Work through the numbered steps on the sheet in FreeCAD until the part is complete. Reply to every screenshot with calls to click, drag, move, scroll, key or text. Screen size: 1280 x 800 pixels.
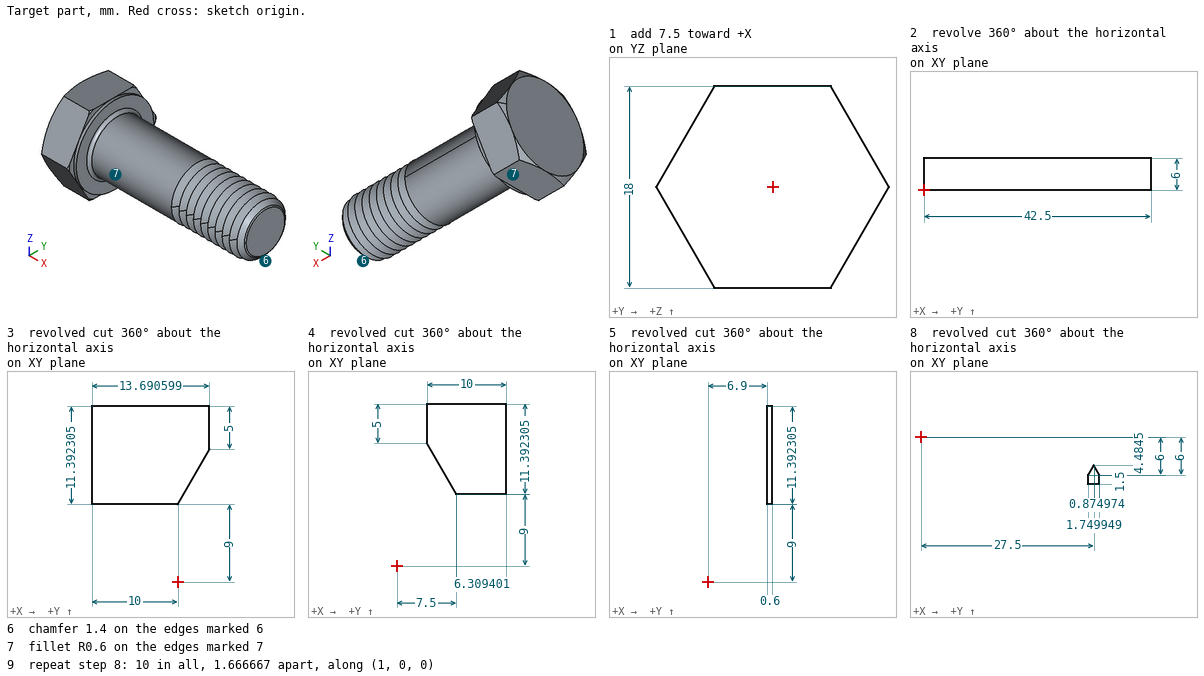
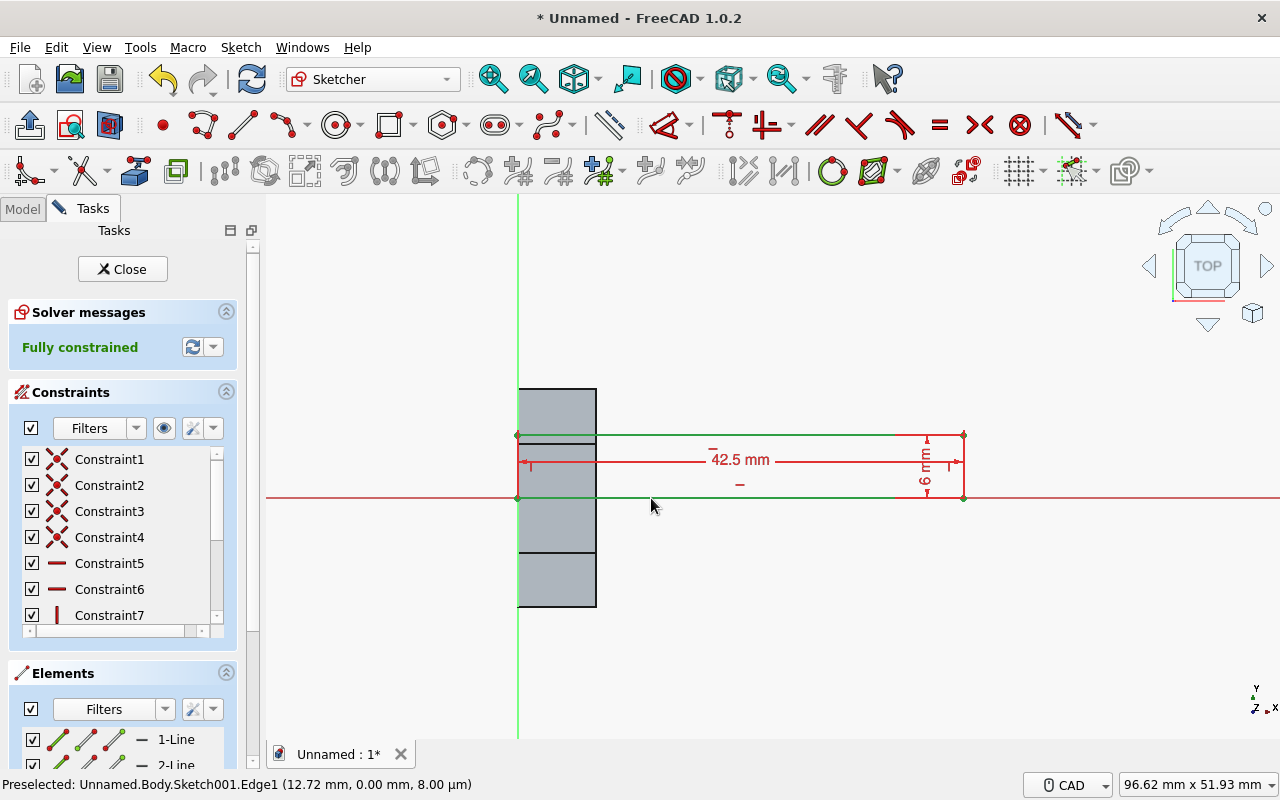
click(123, 269)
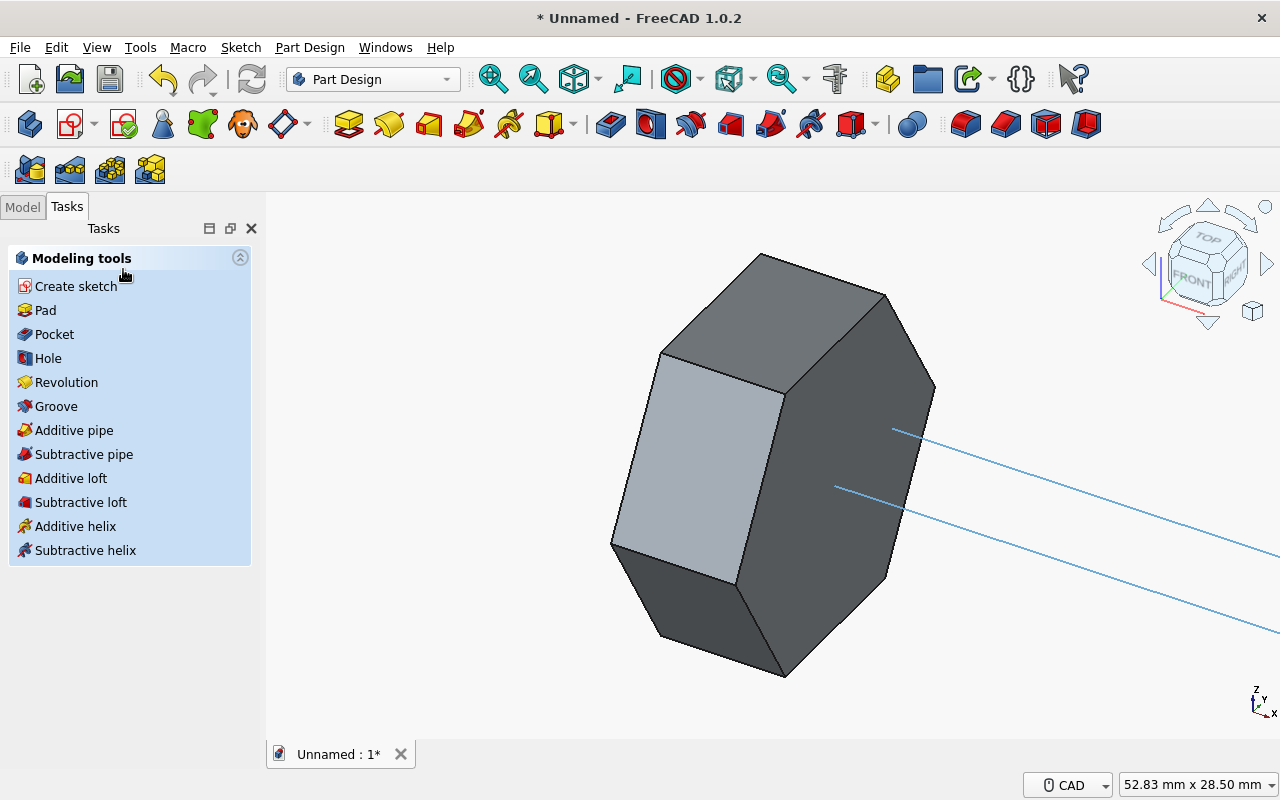
click(390, 124)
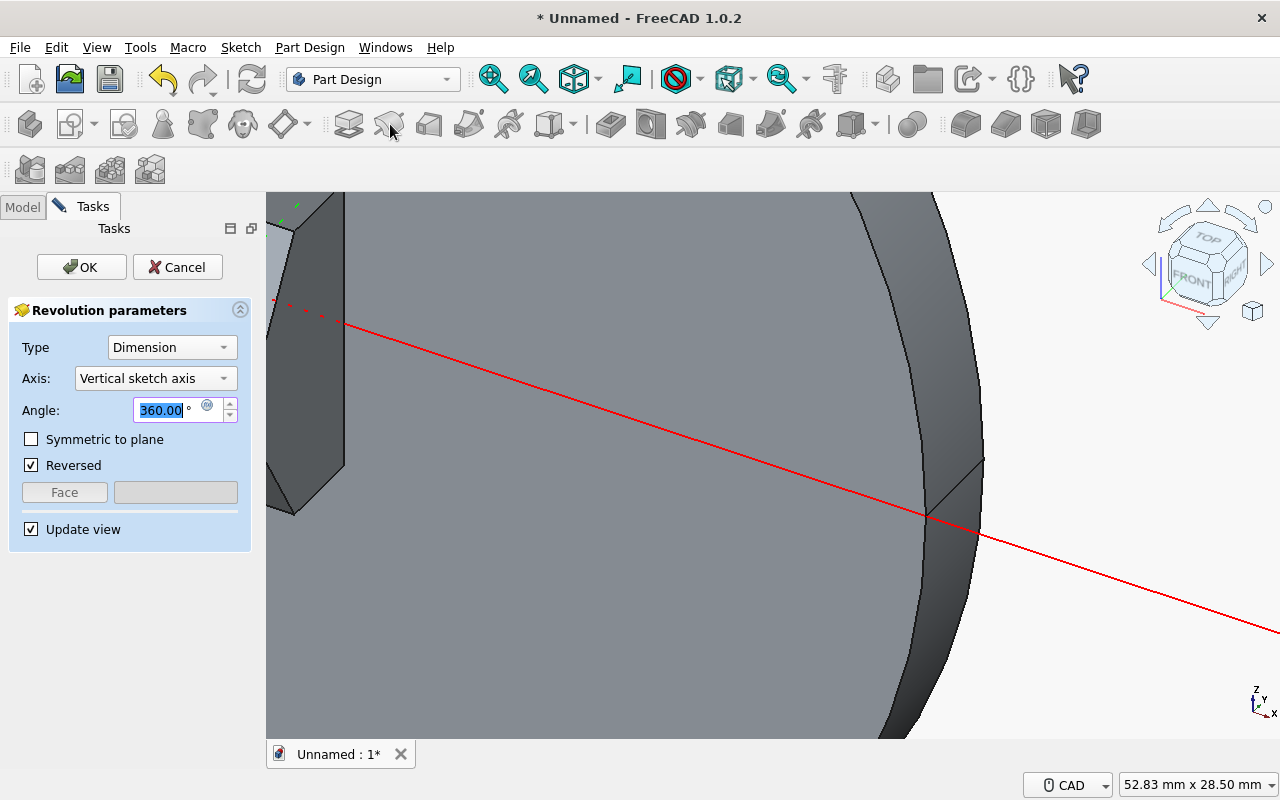
click(156, 378)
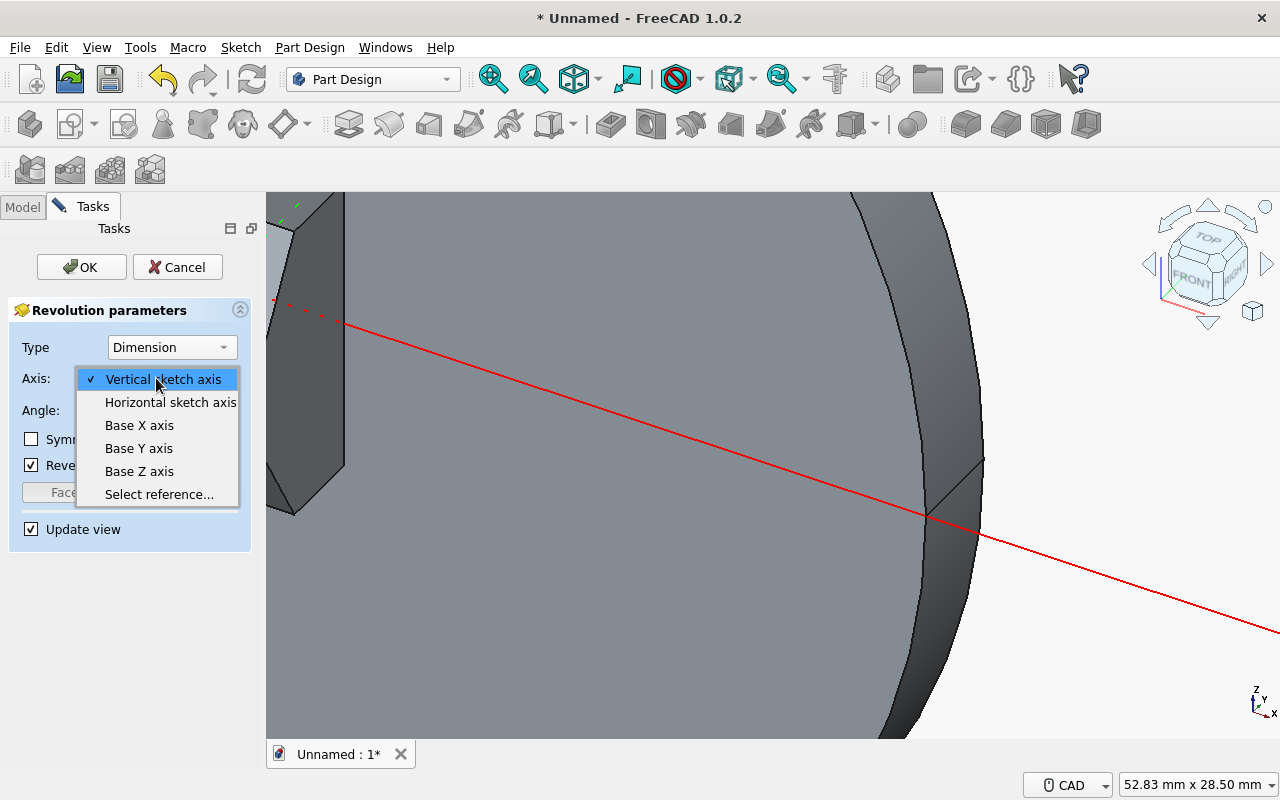
click(156, 402)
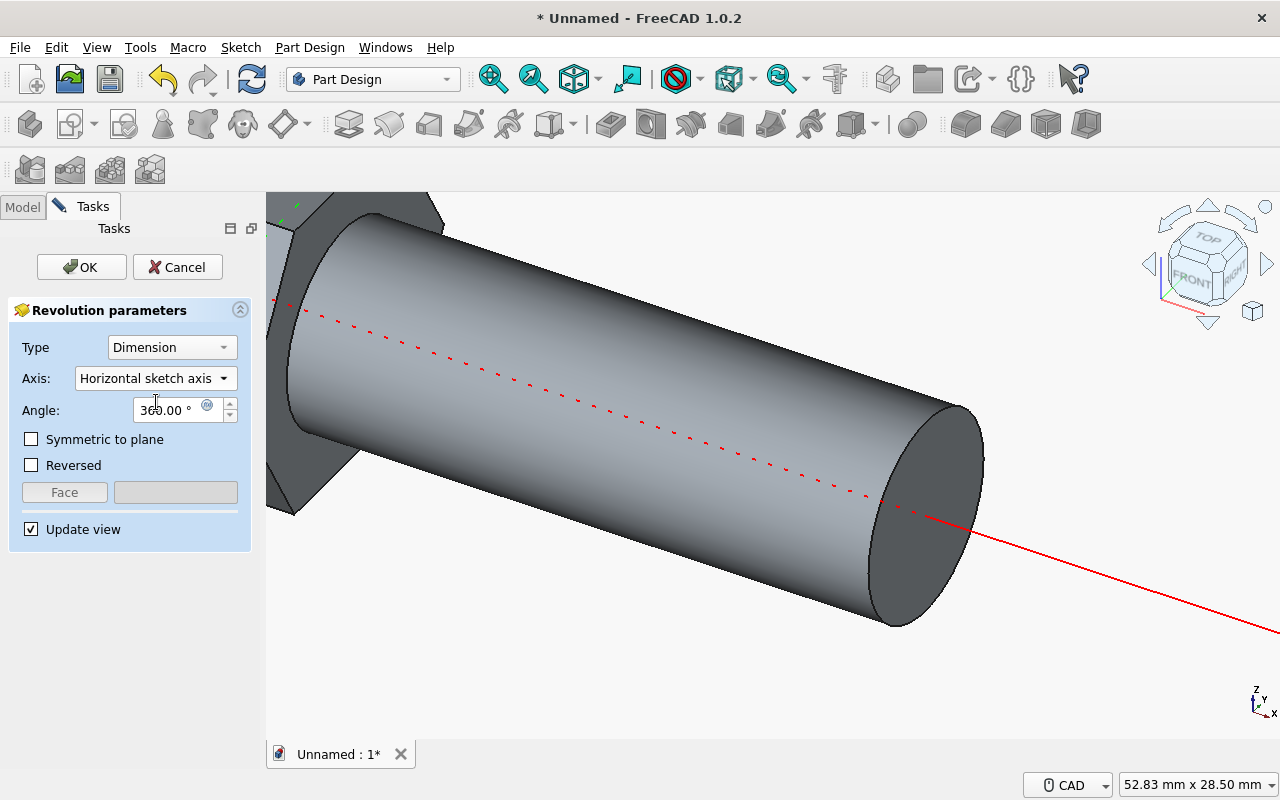
click(82, 267)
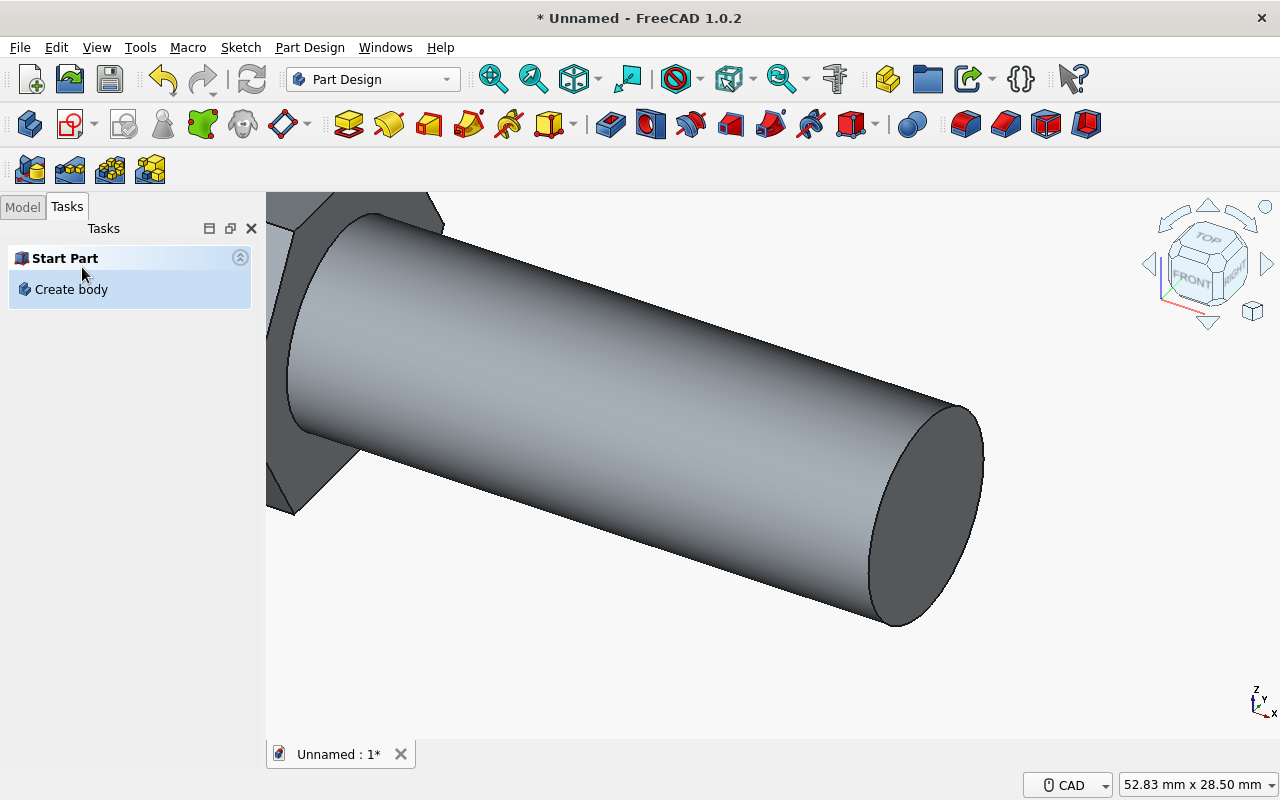
key(v)
key(f)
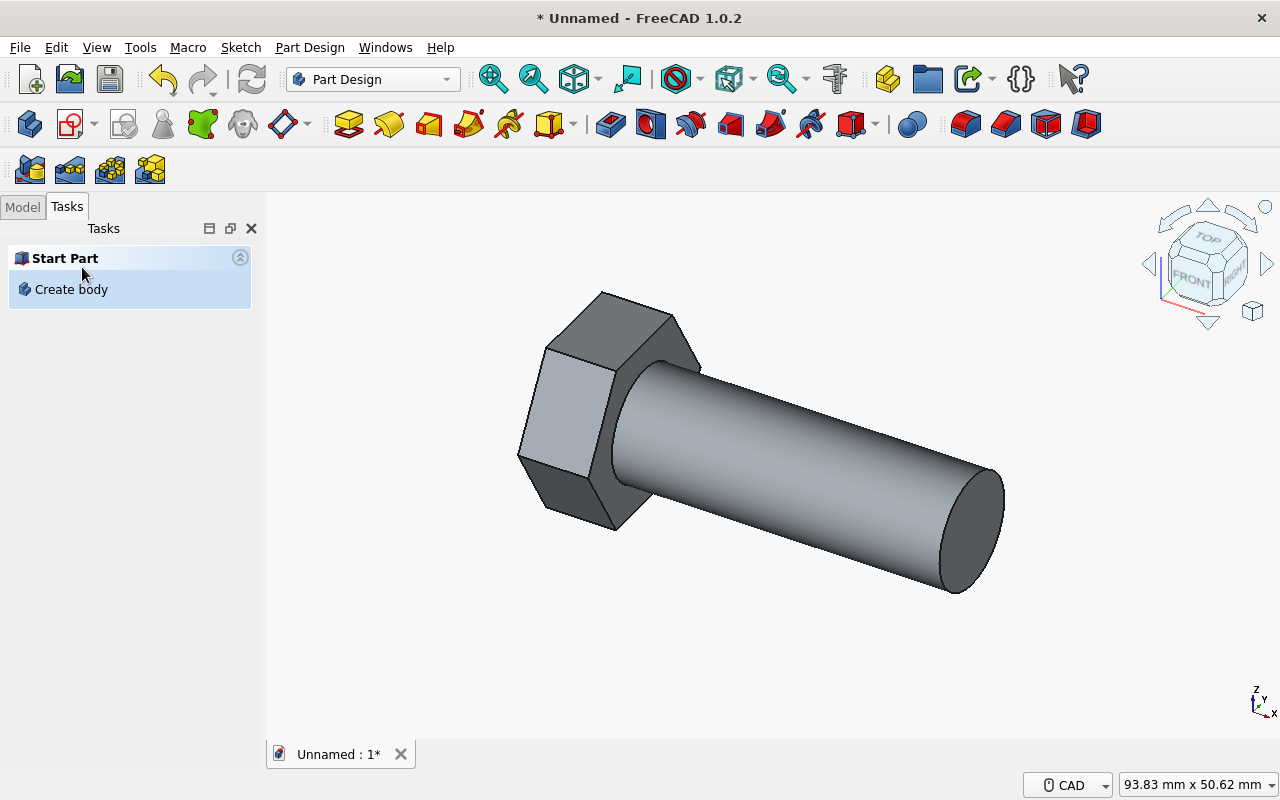
click(70, 124)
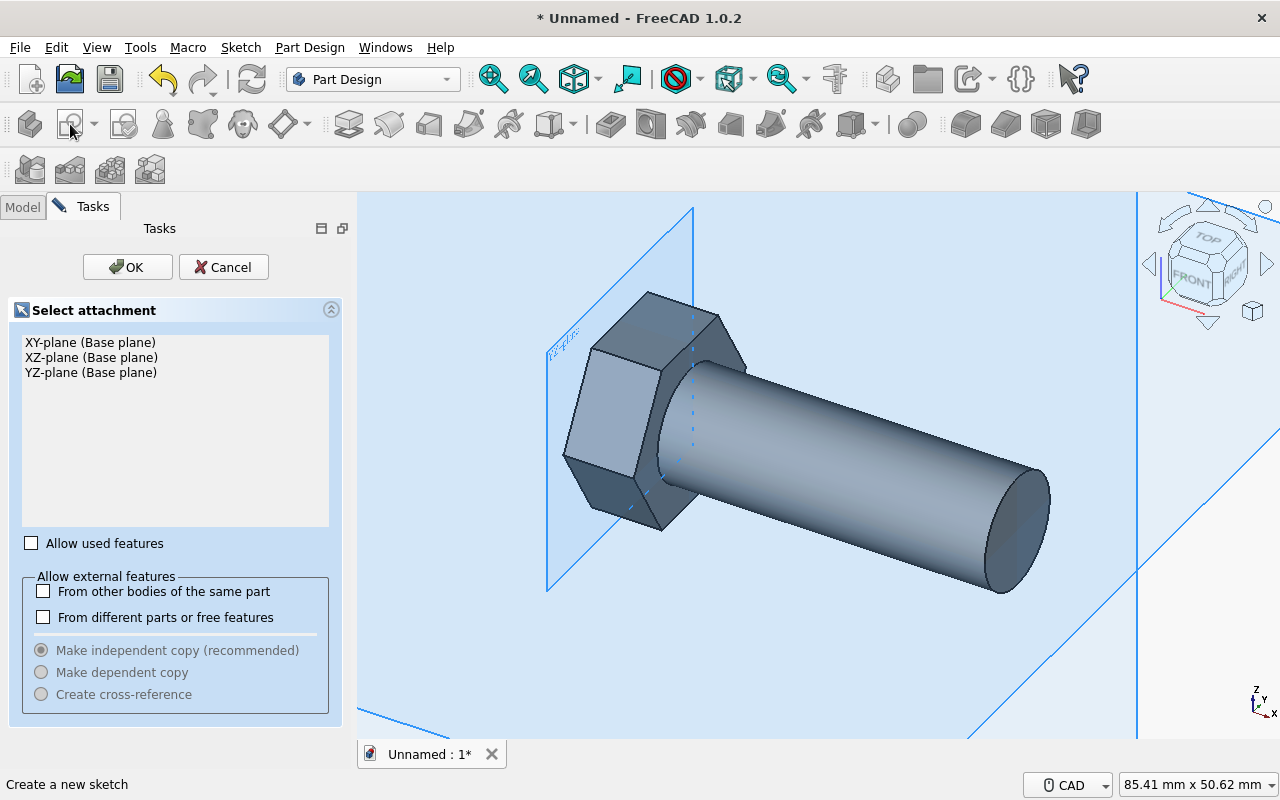
click(82, 342)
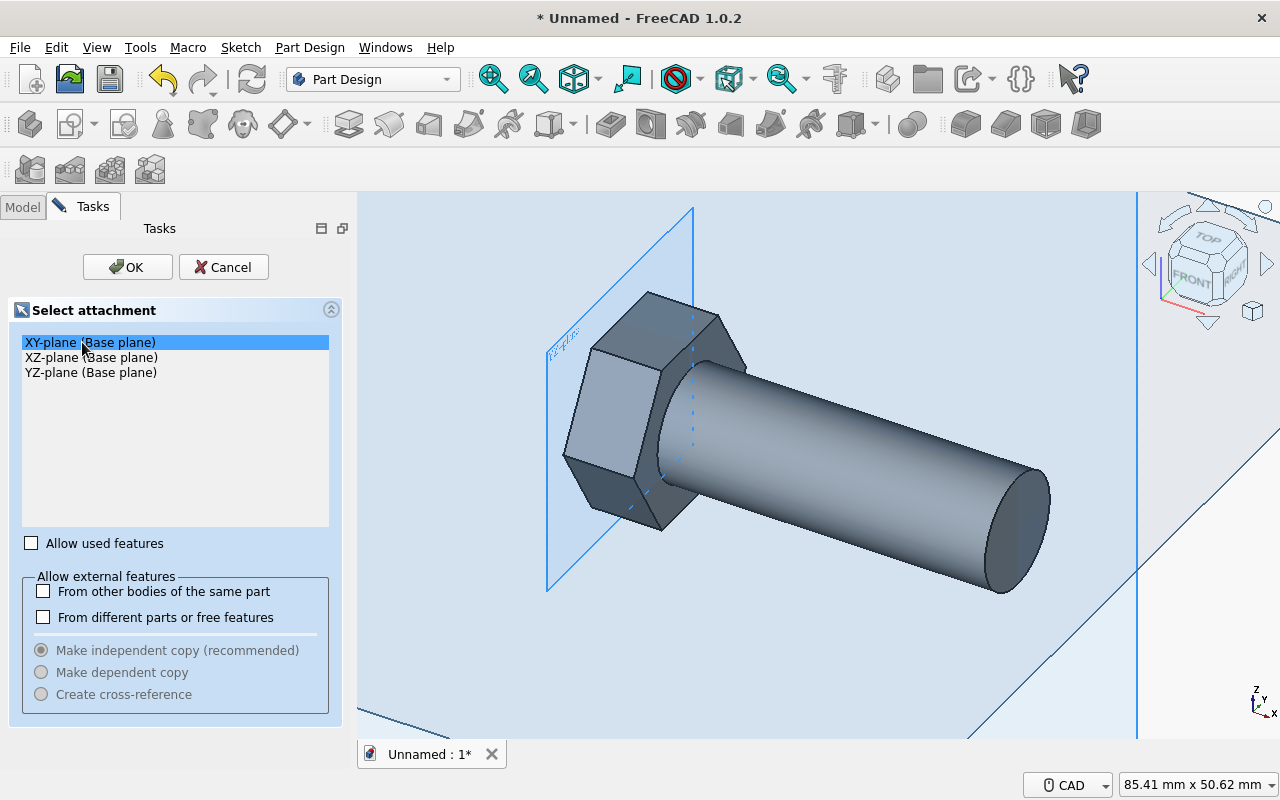
click(128, 267)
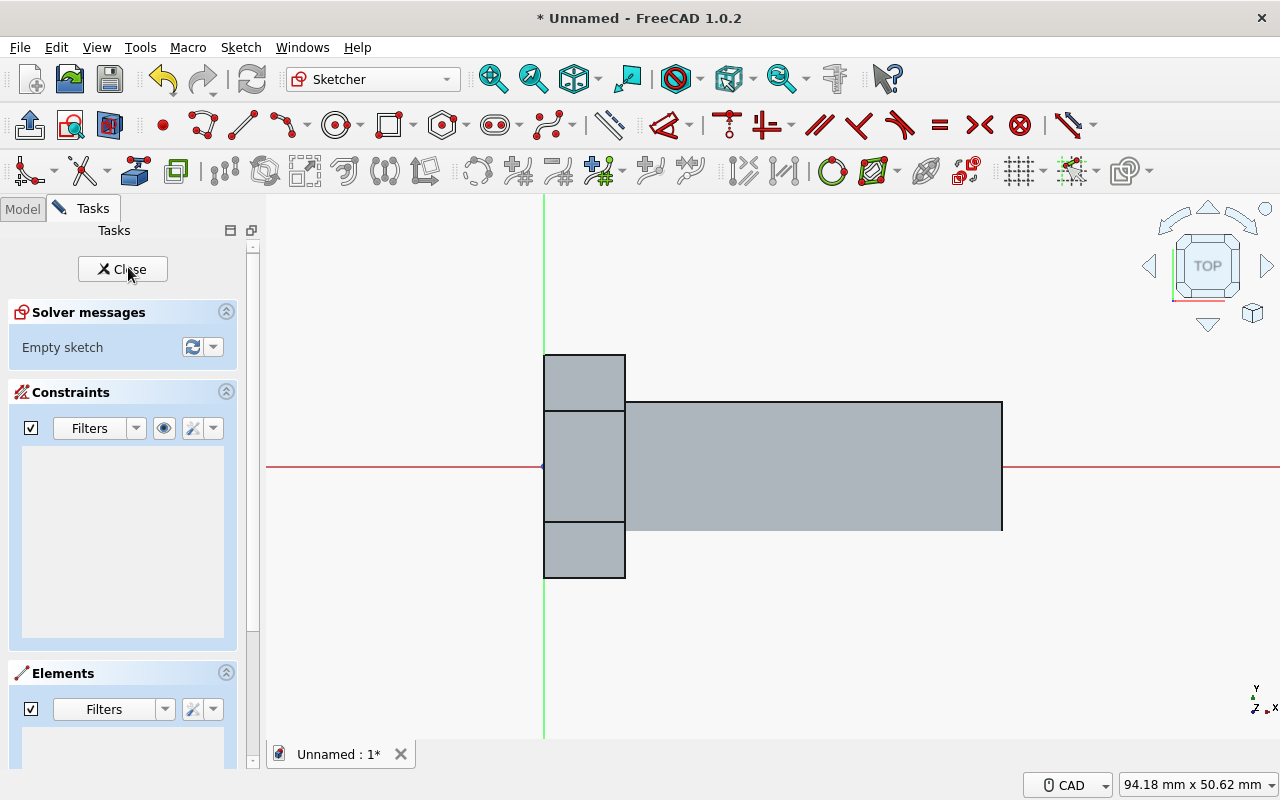
key(q)
key(s)